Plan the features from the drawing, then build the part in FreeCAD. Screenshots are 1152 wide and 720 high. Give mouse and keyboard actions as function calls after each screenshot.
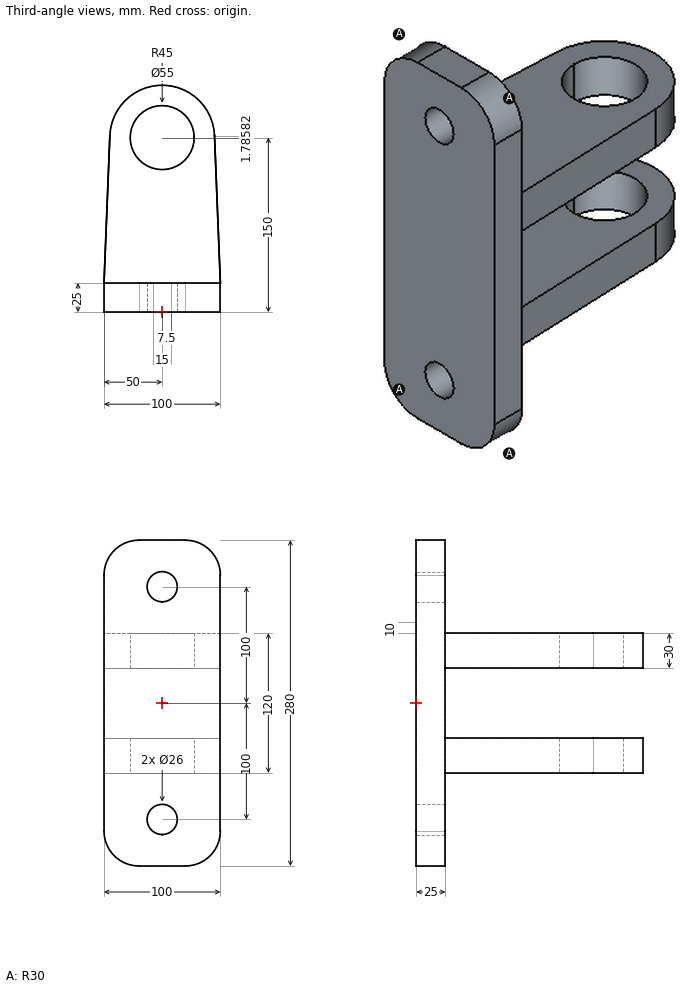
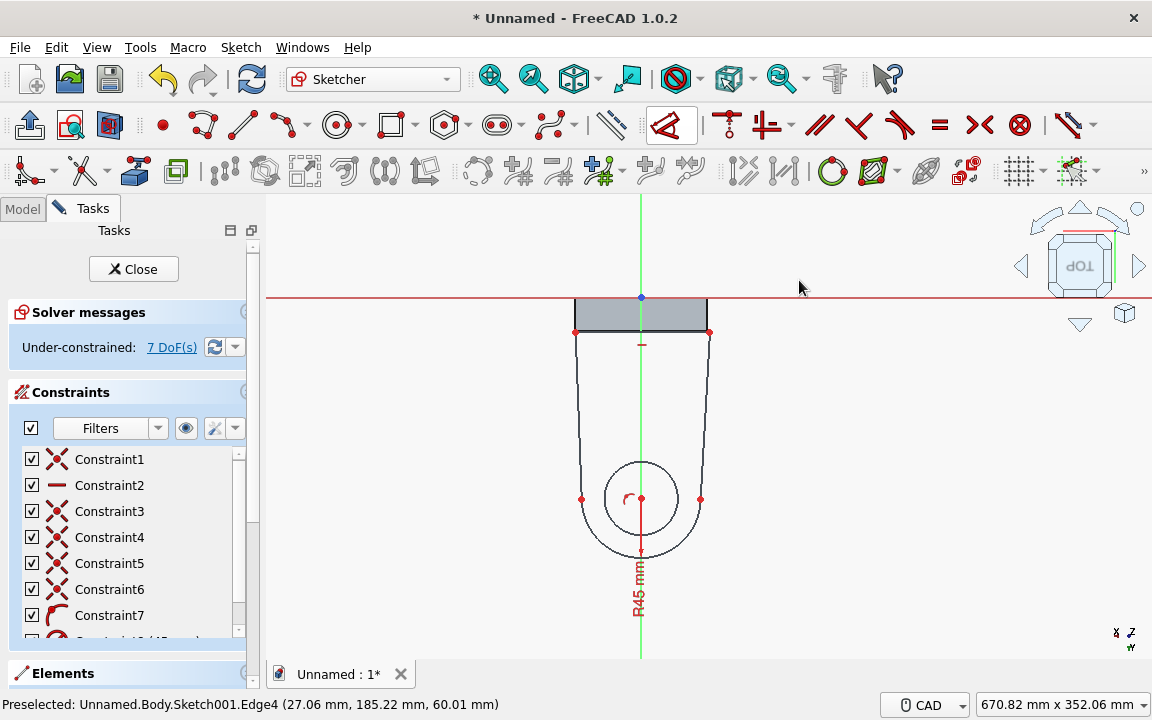
click(667, 473)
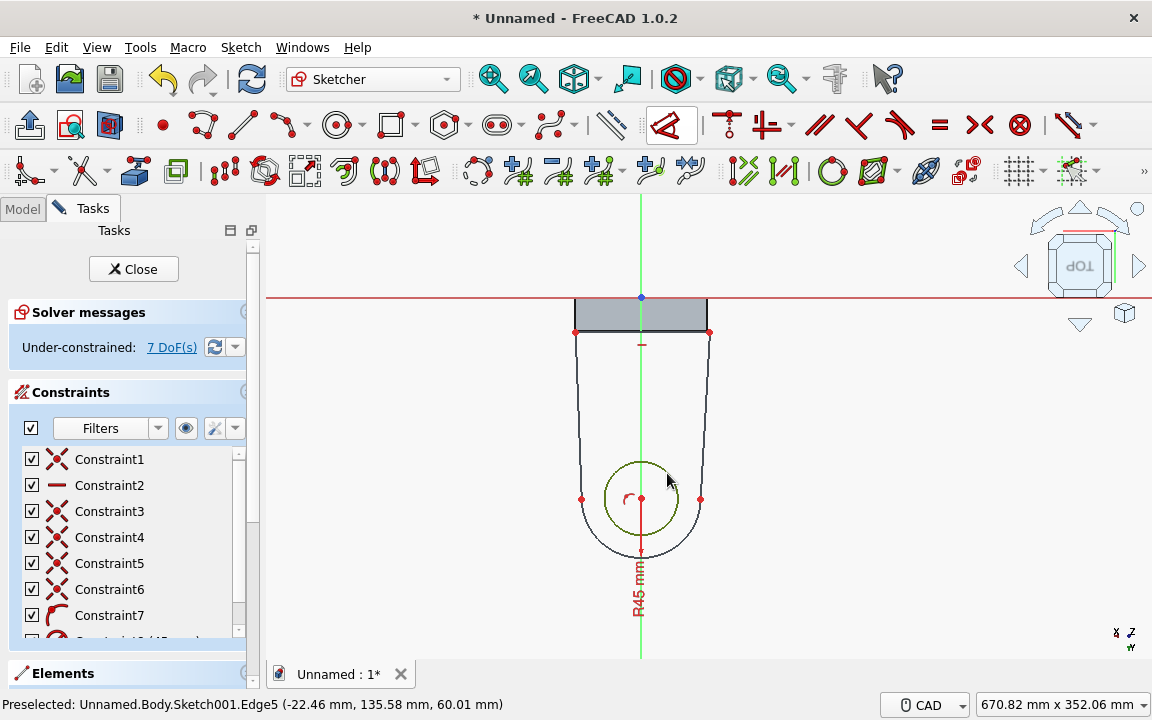
click(692, 126)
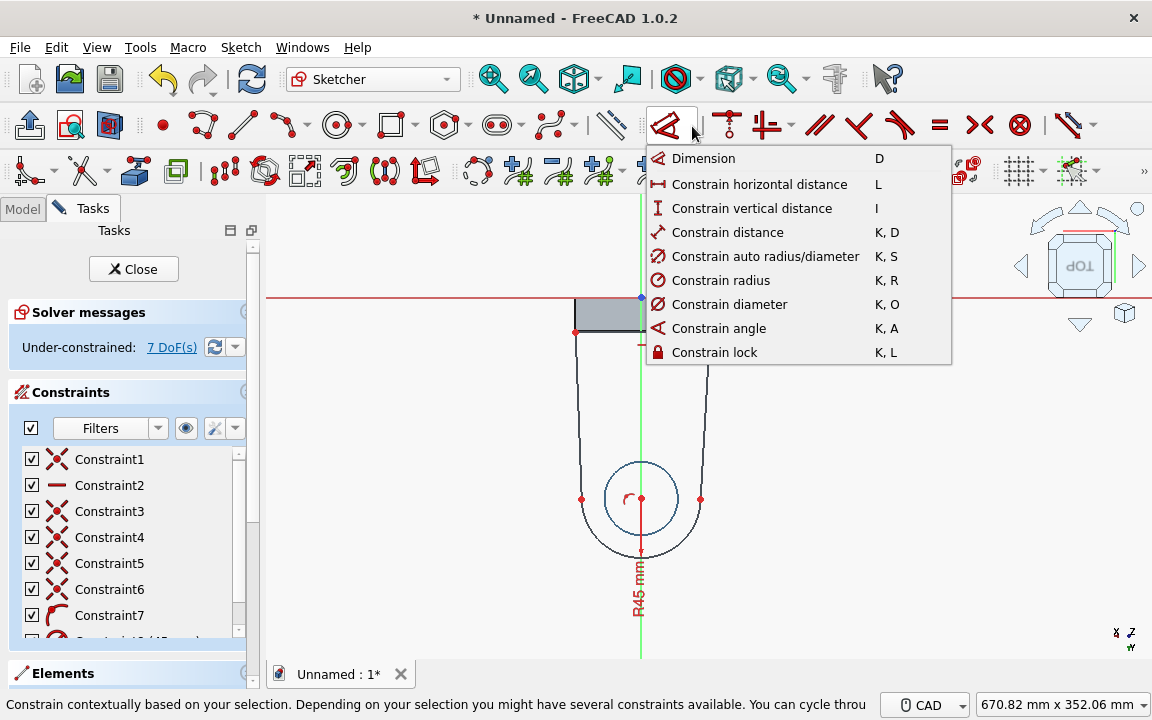
click(799, 304)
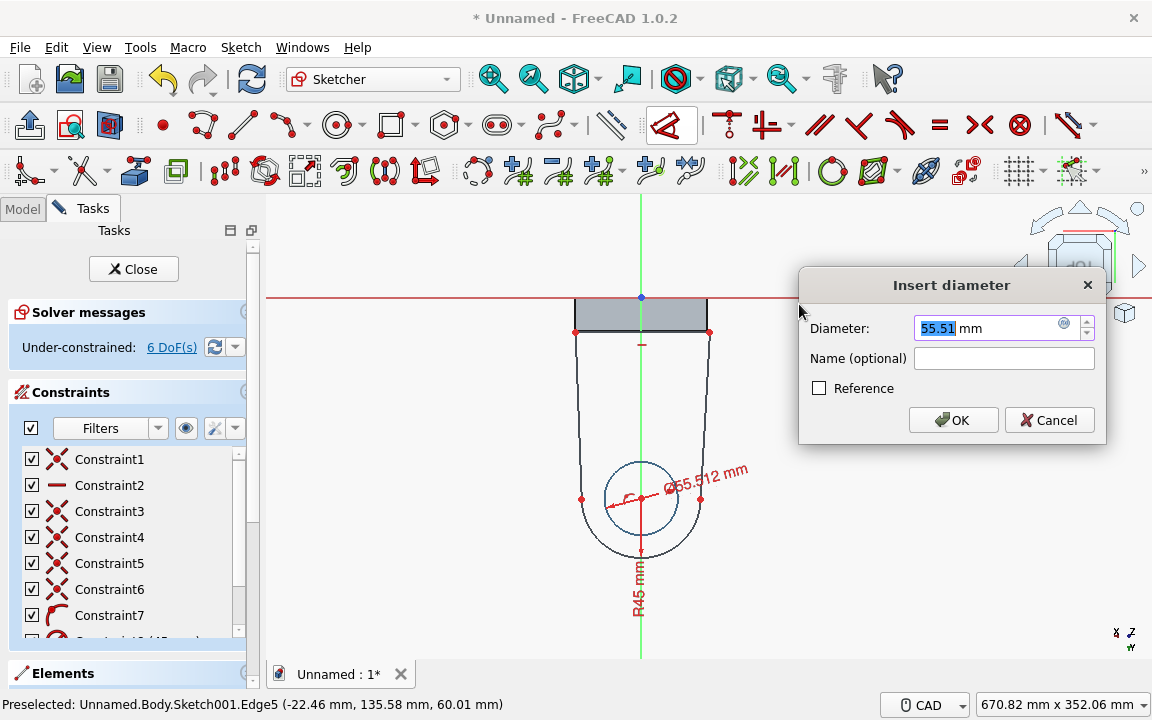
text(55)
key(Return)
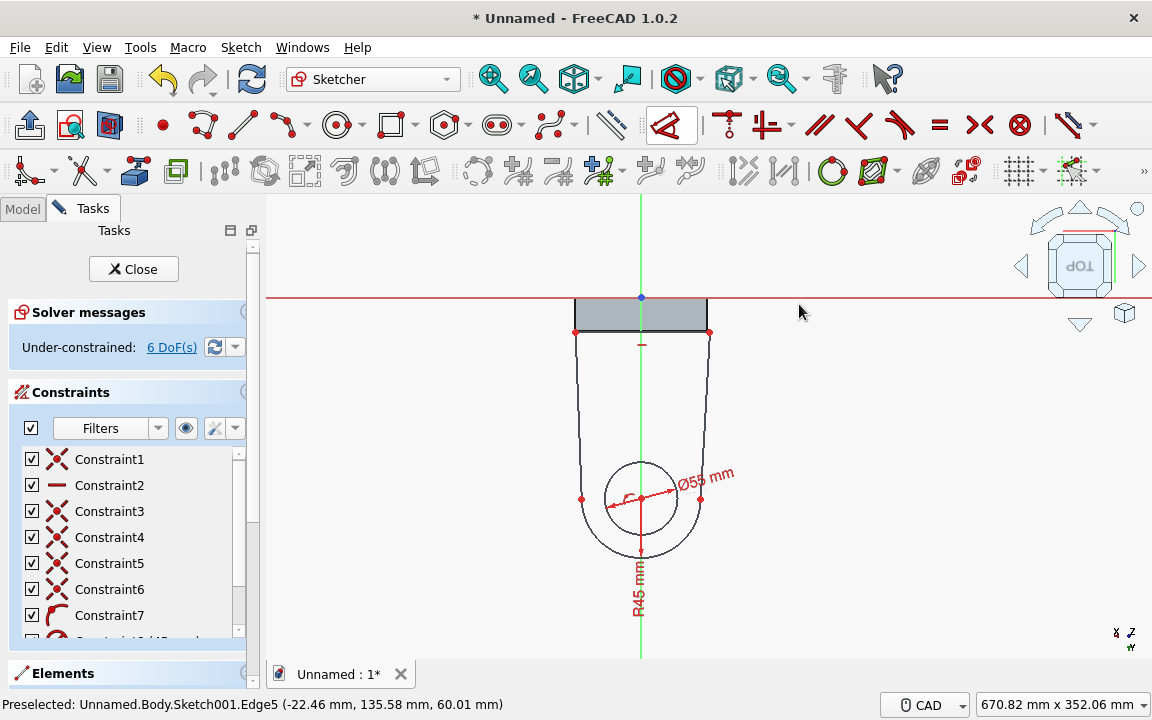
click(670, 332)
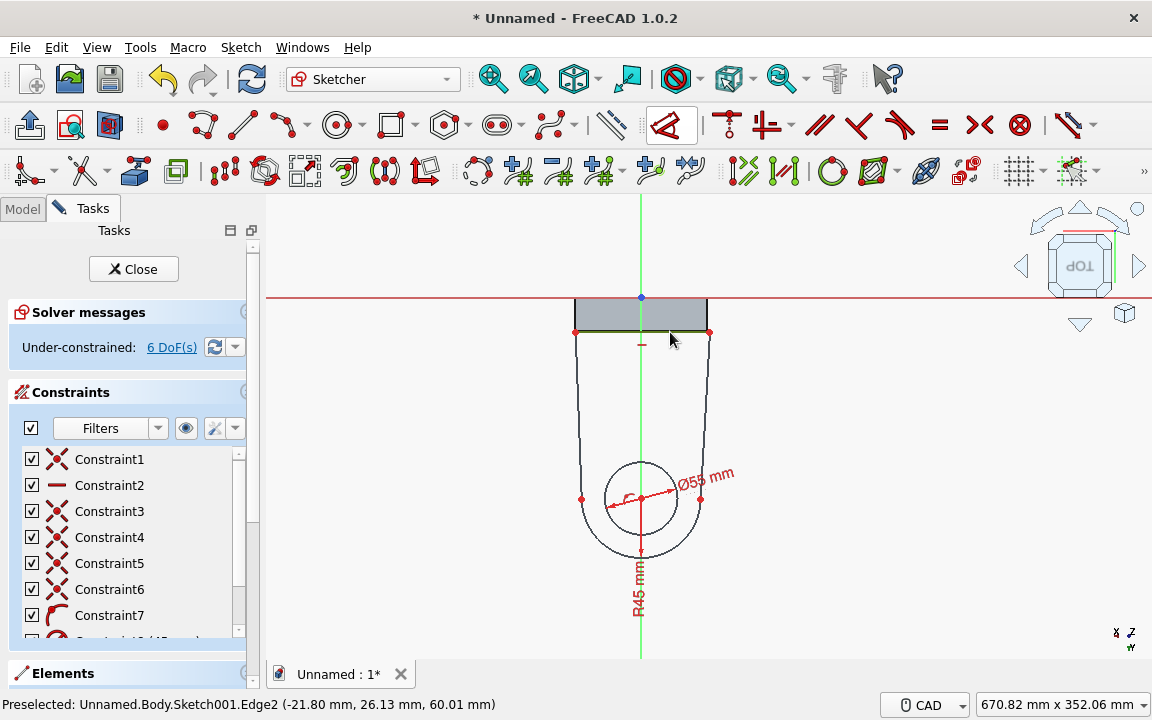
click(692, 126)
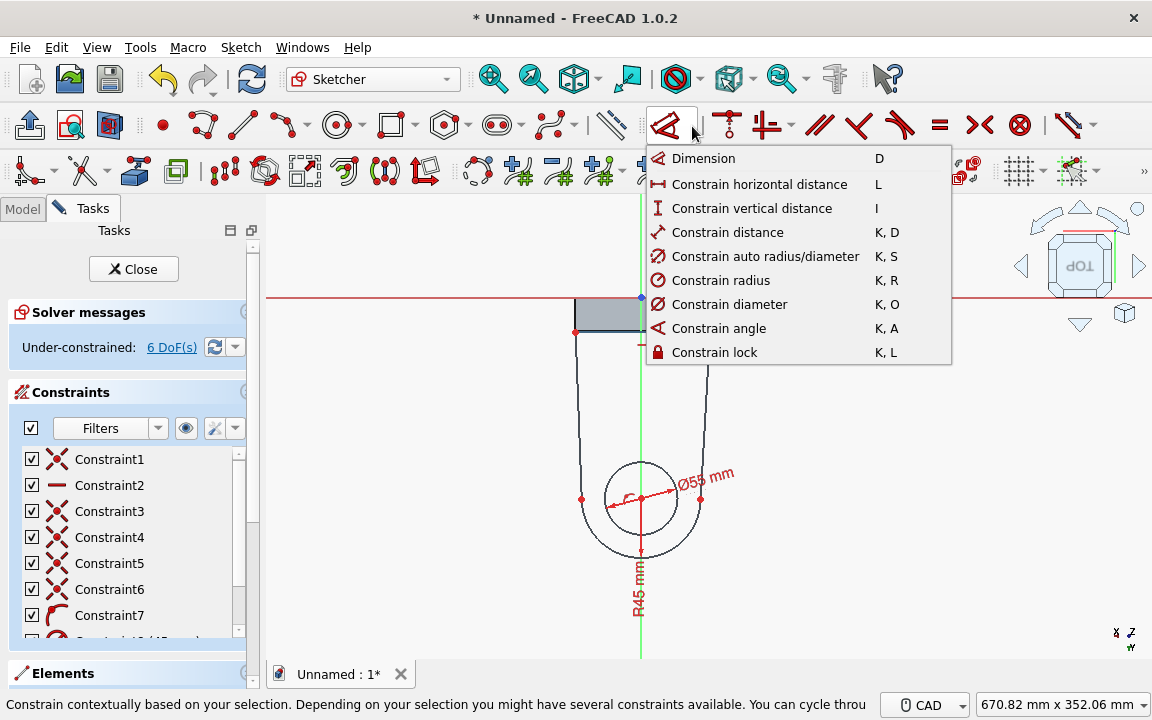
click(799, 184)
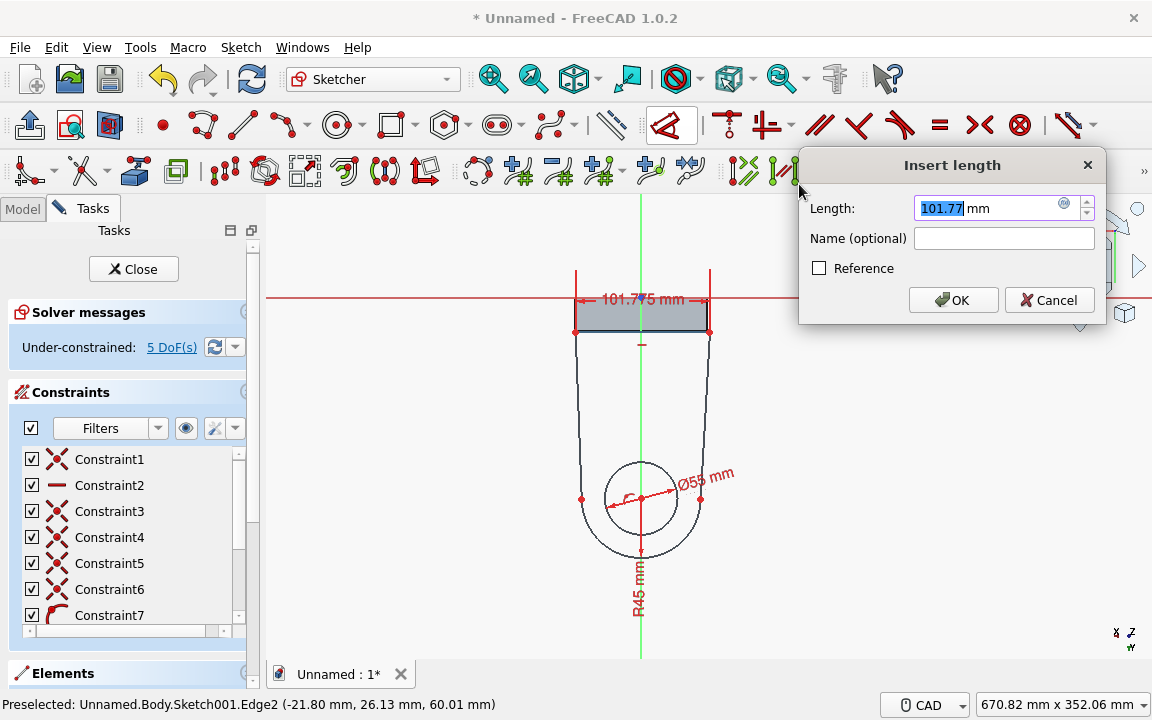
text(100)
key(Return)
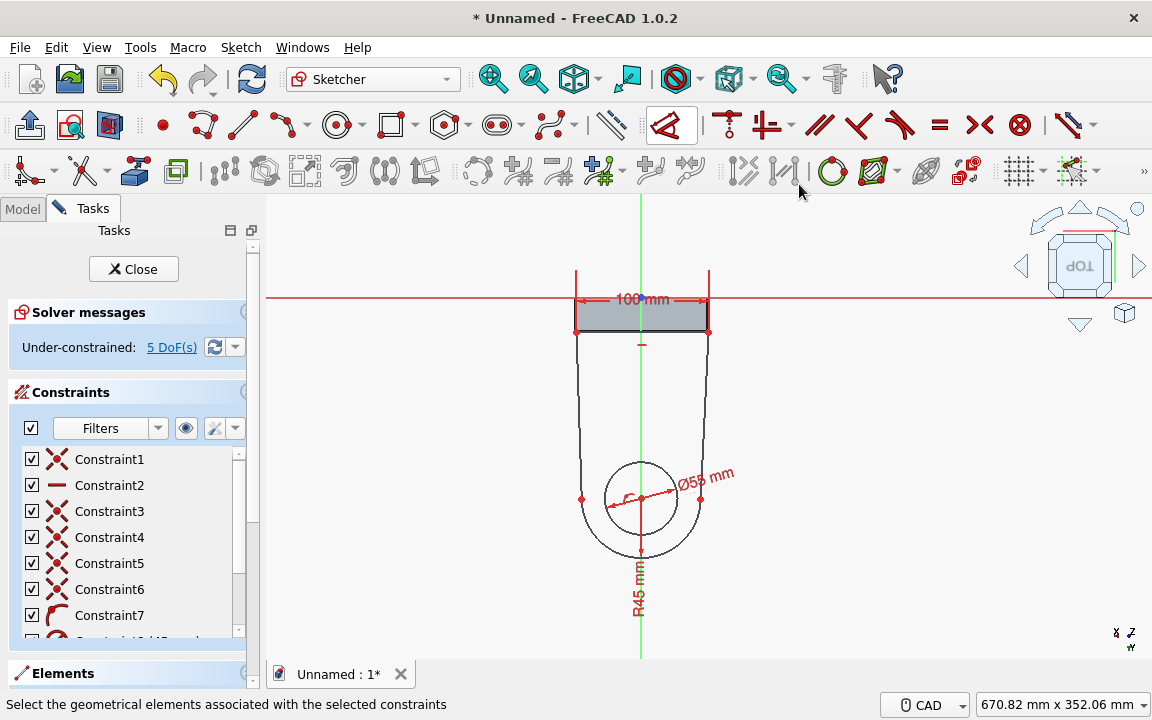
click(709, 332)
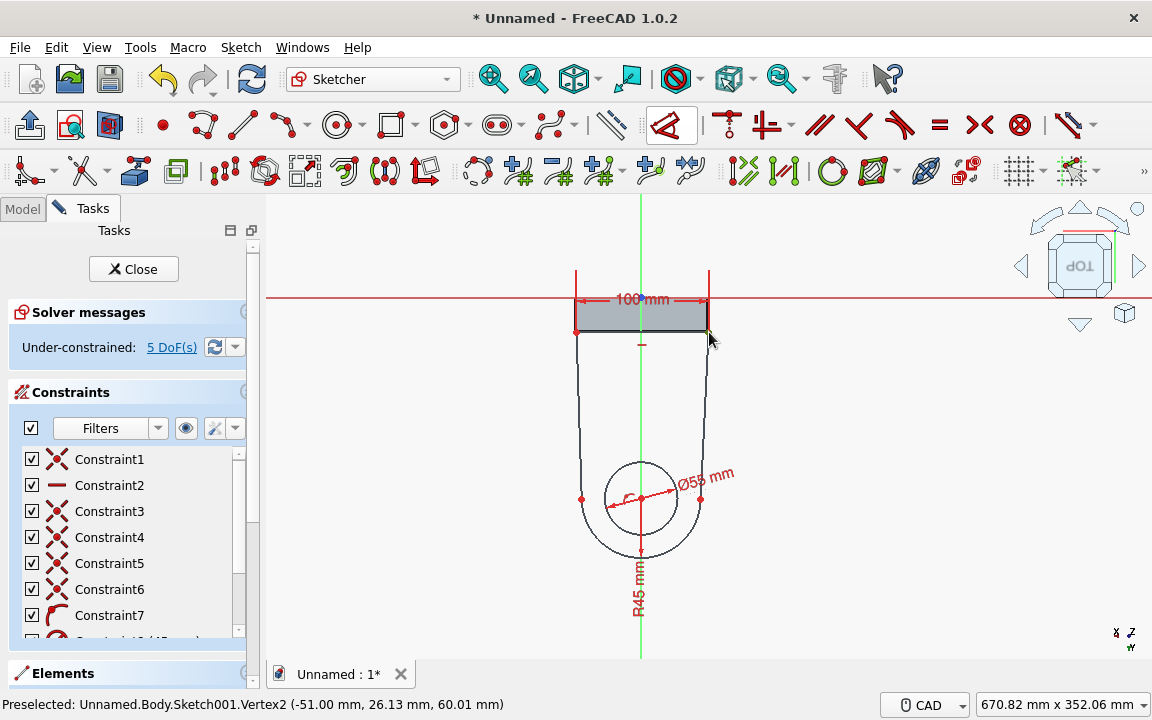
click(692, 126)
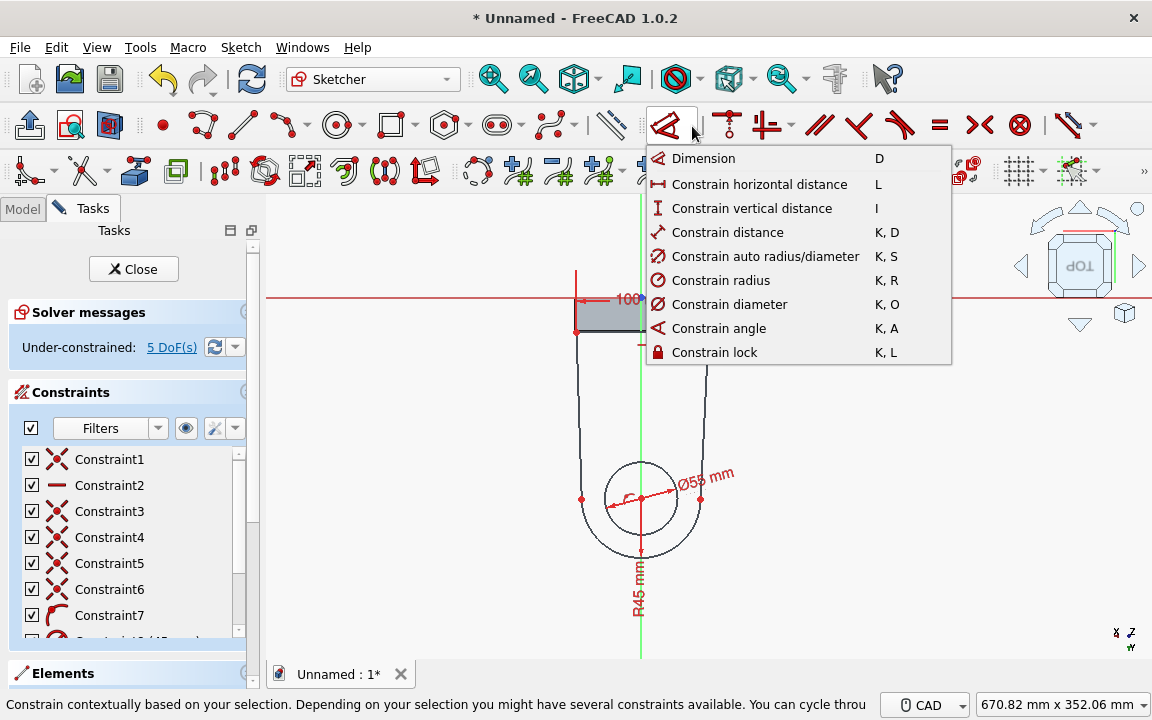
click(799, 184)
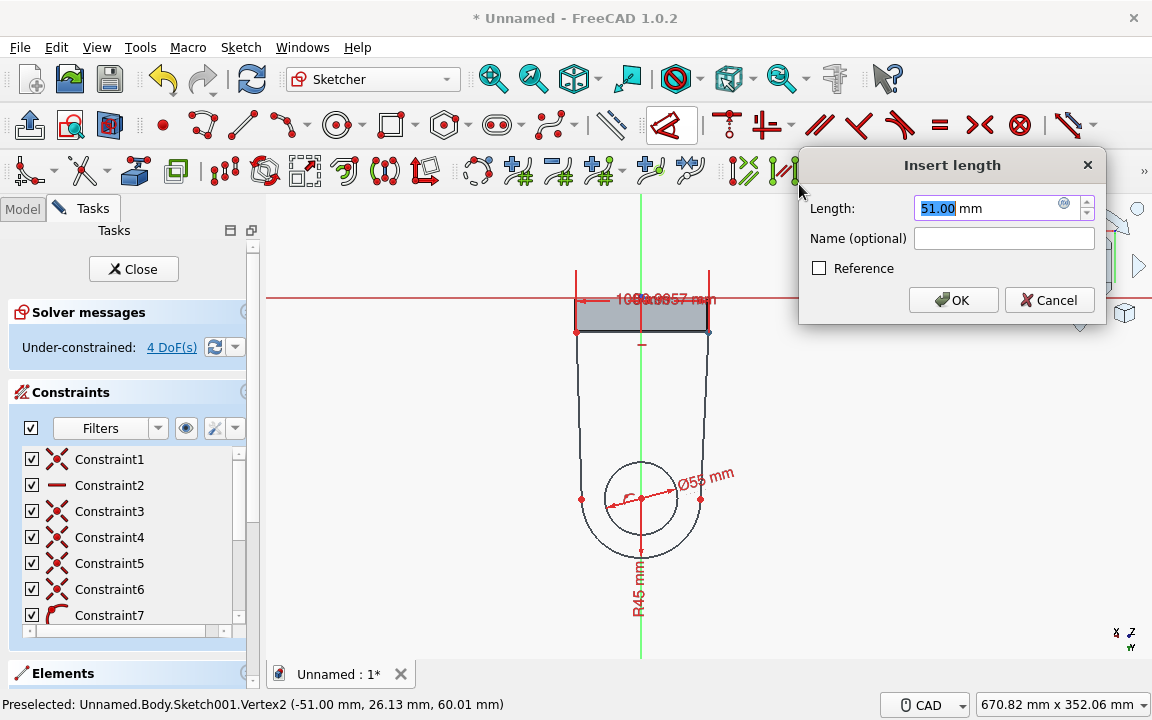
text(50)
key(Return)